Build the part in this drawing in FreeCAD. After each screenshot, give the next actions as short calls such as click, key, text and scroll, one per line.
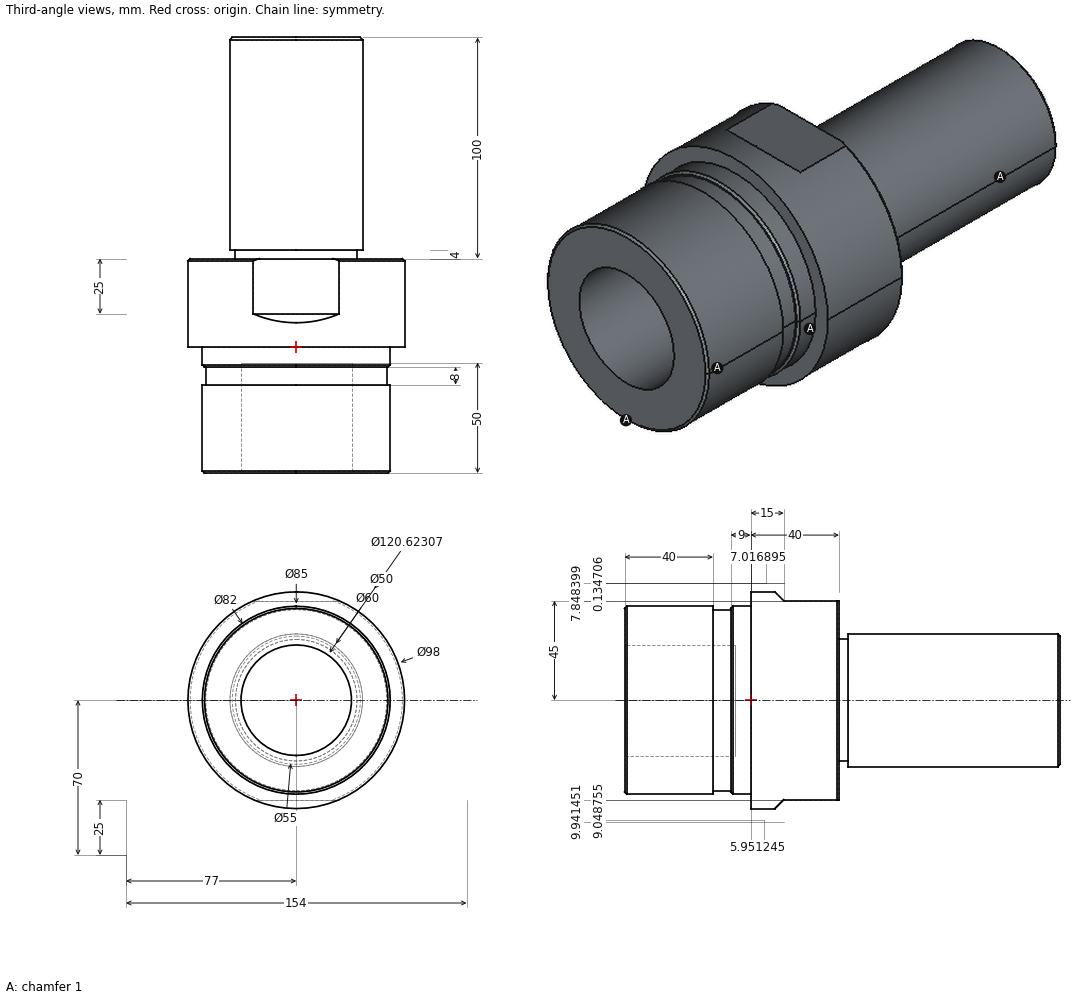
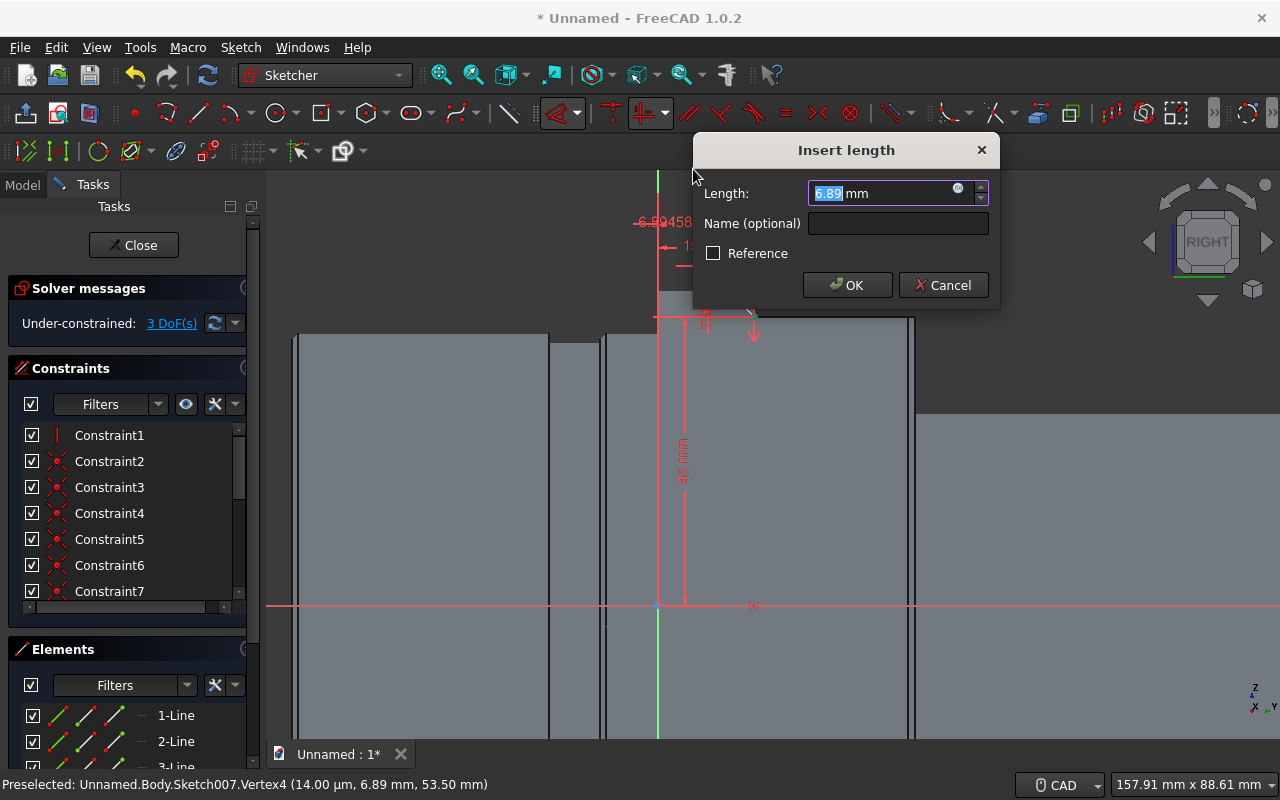
text(7.016895)
key(Return)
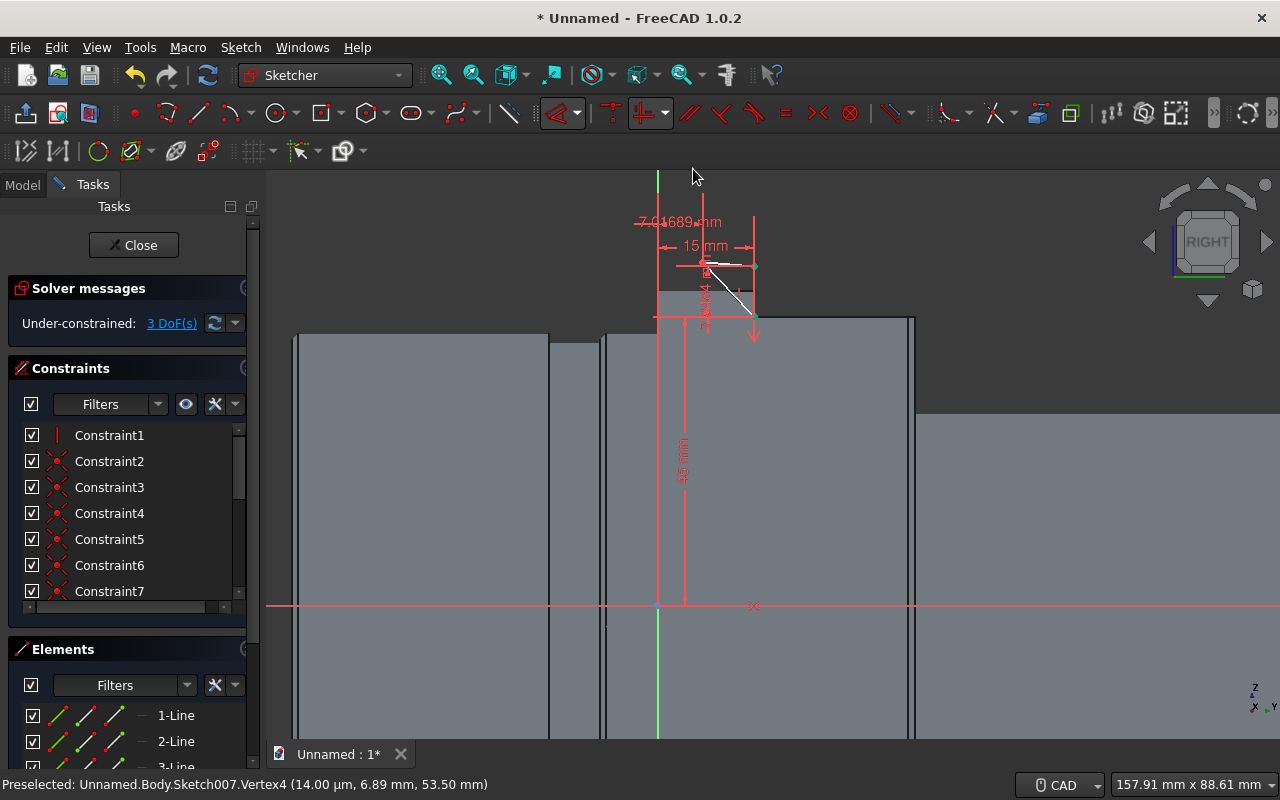
scroll(703, 263, down, 3)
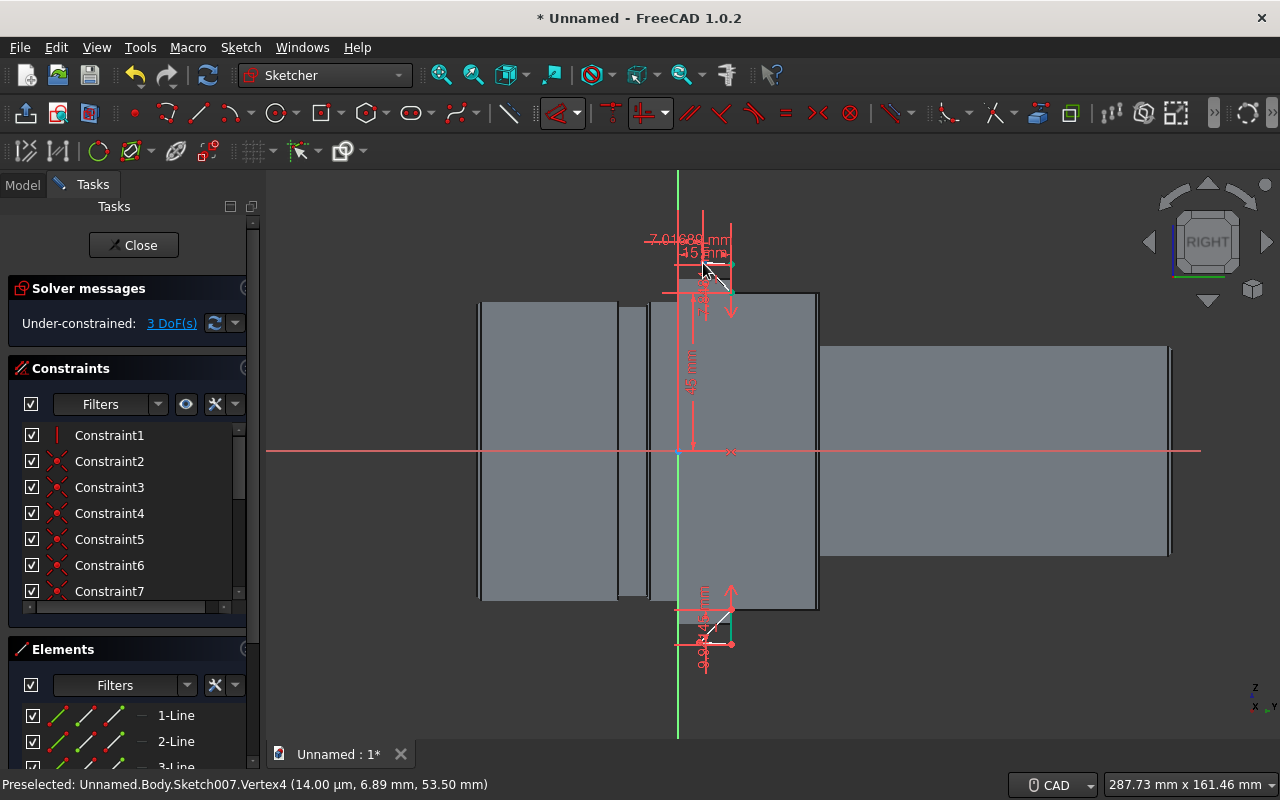
scroll(700, 643, up, 4)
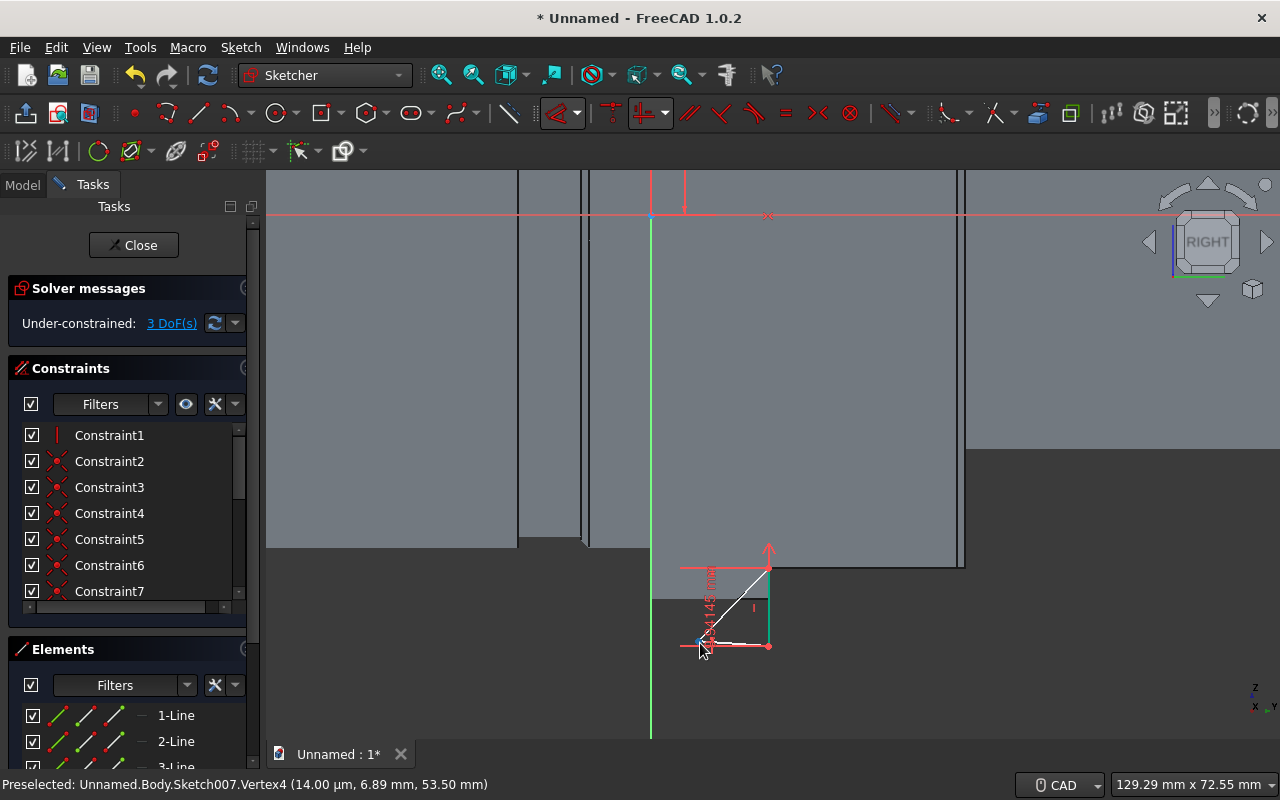
click(699, 641)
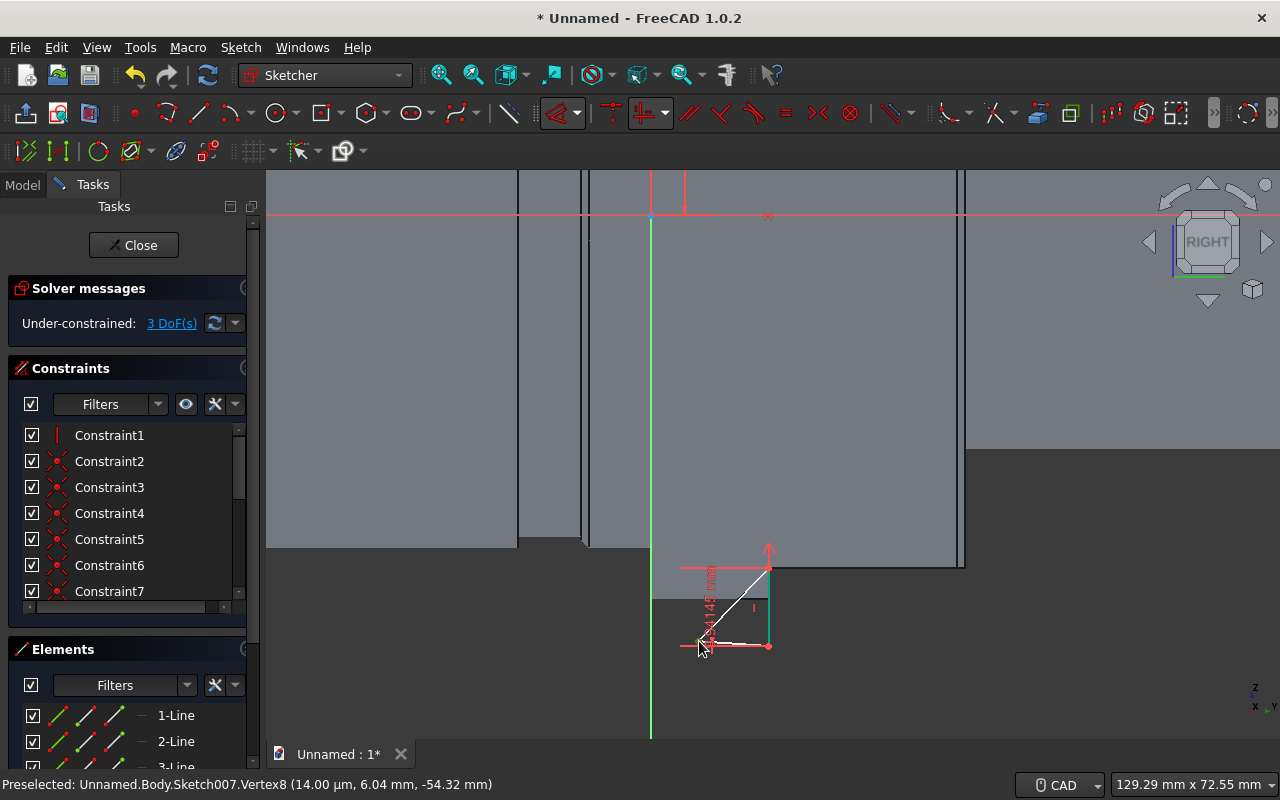
key(l)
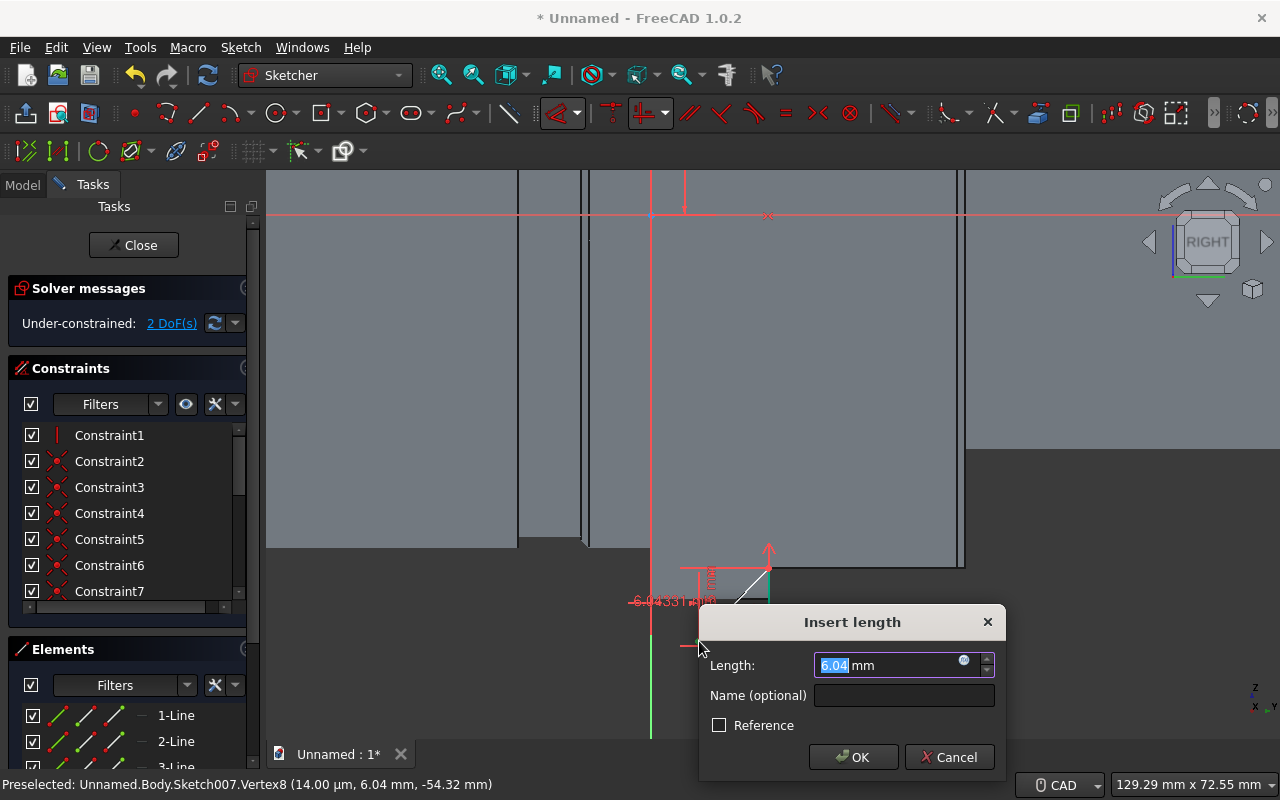
text(5.951245)
key(Return)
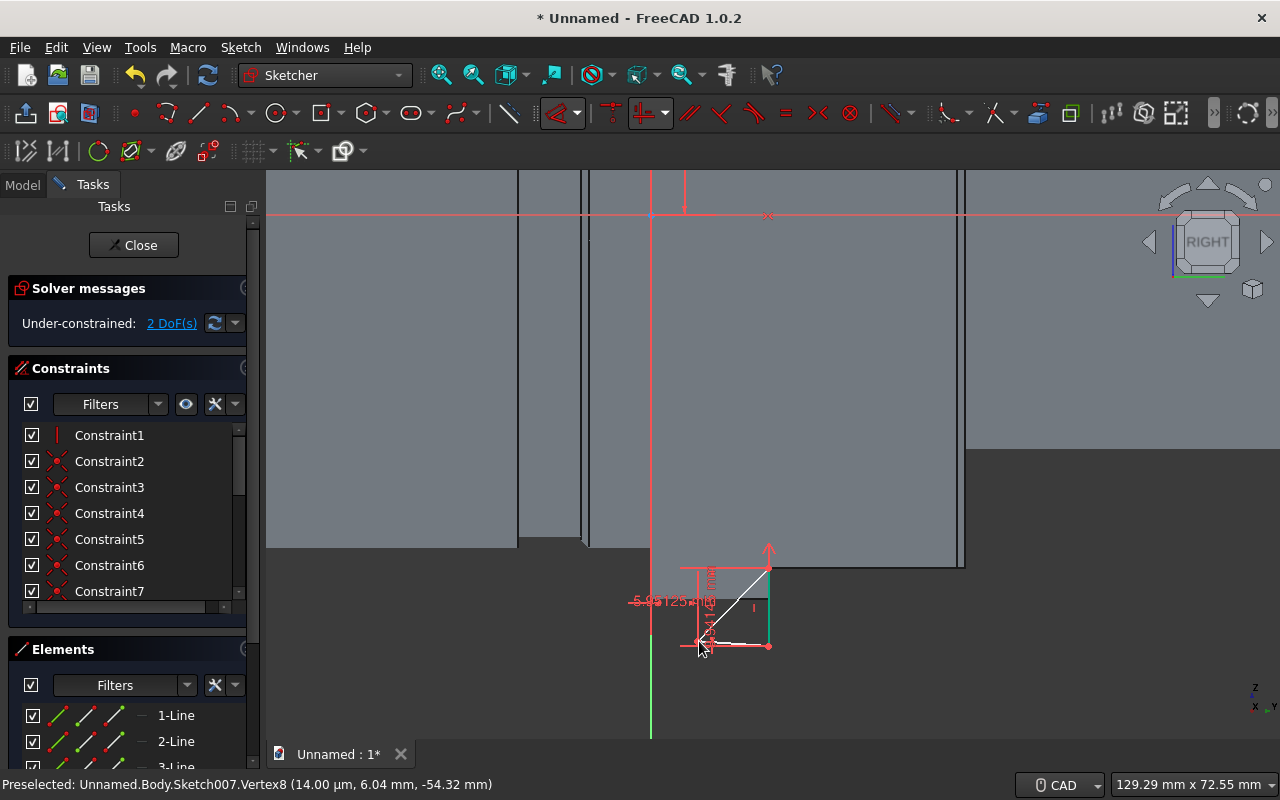
scroll(700, 644, down, 4)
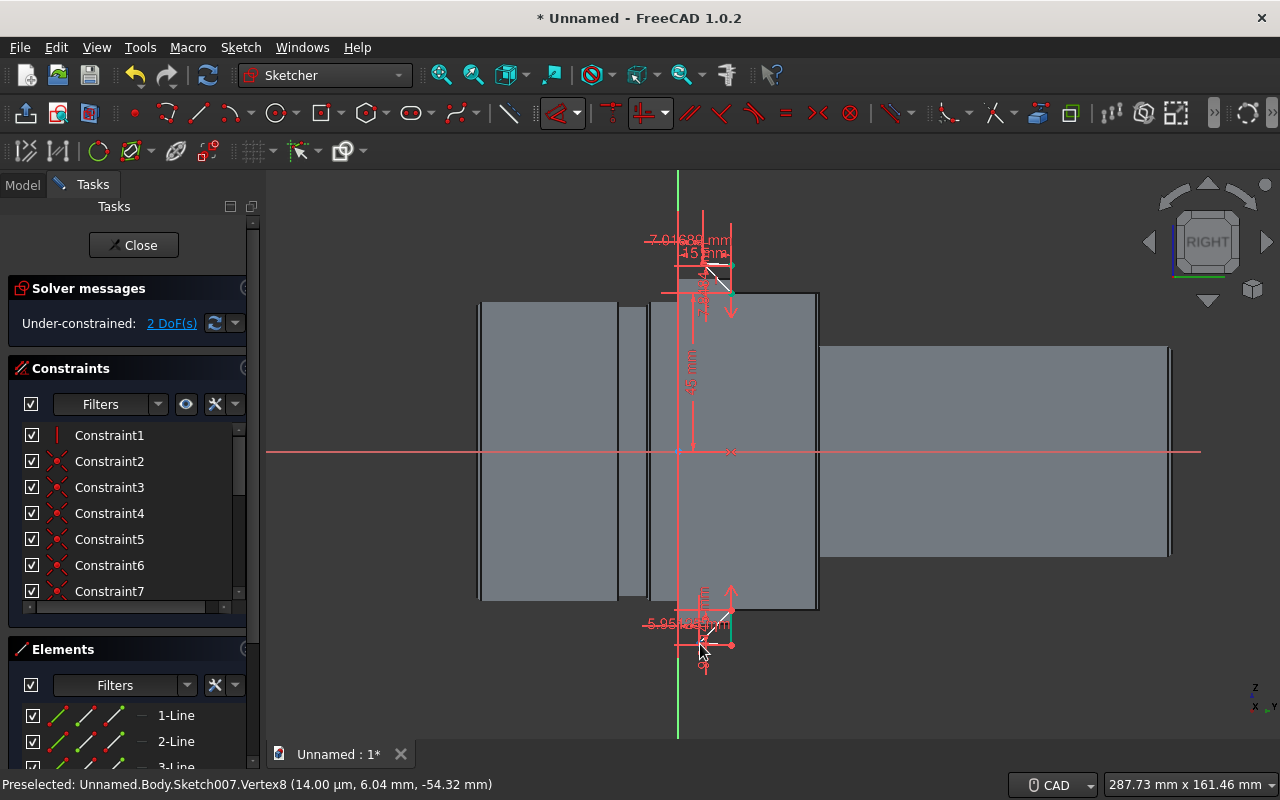
scroll(723, 265, up, 23)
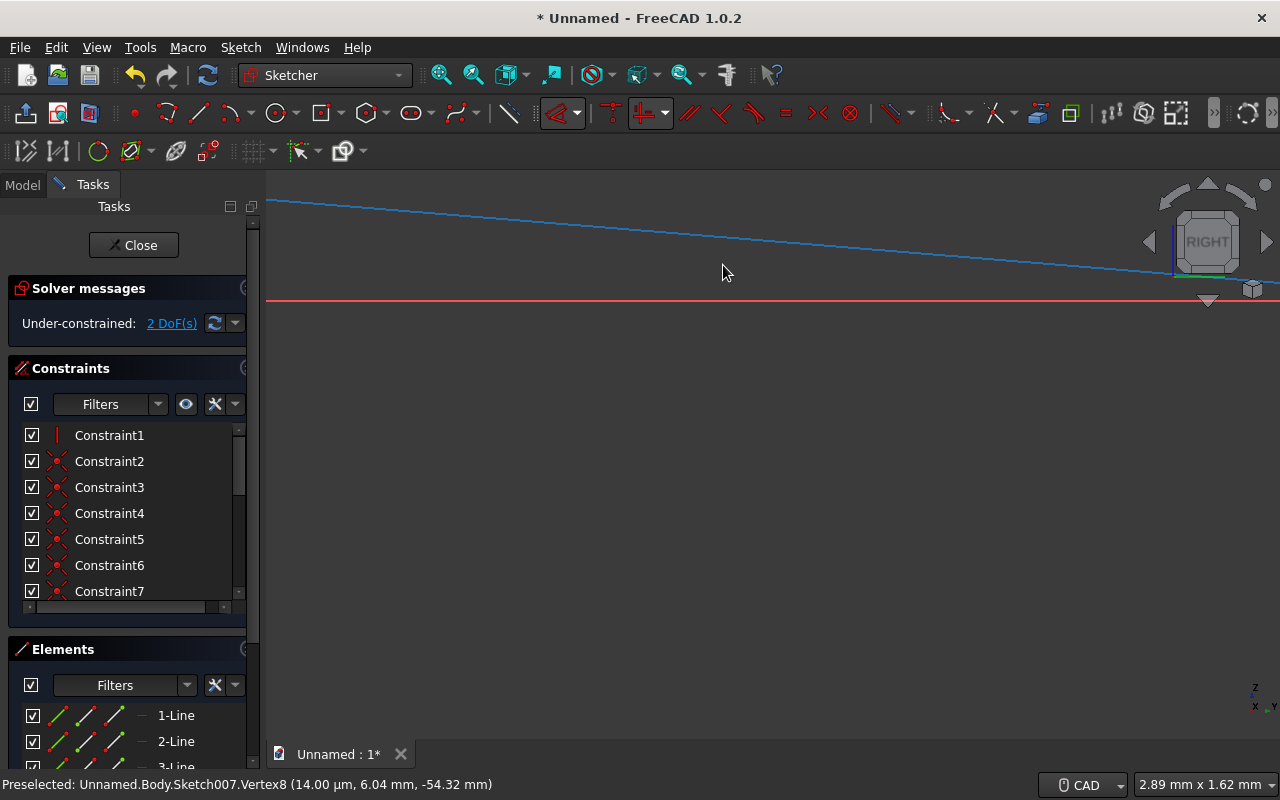
click(657, 232)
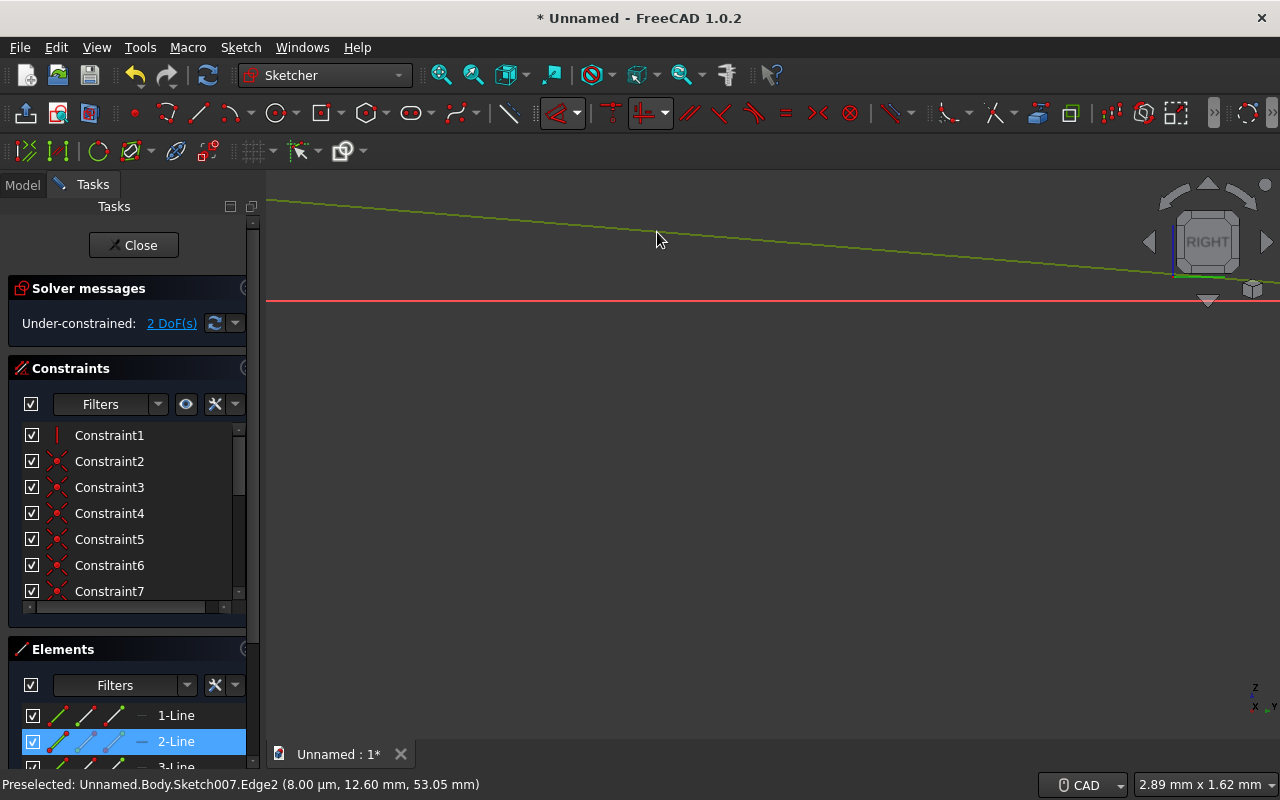
click(580, 114)